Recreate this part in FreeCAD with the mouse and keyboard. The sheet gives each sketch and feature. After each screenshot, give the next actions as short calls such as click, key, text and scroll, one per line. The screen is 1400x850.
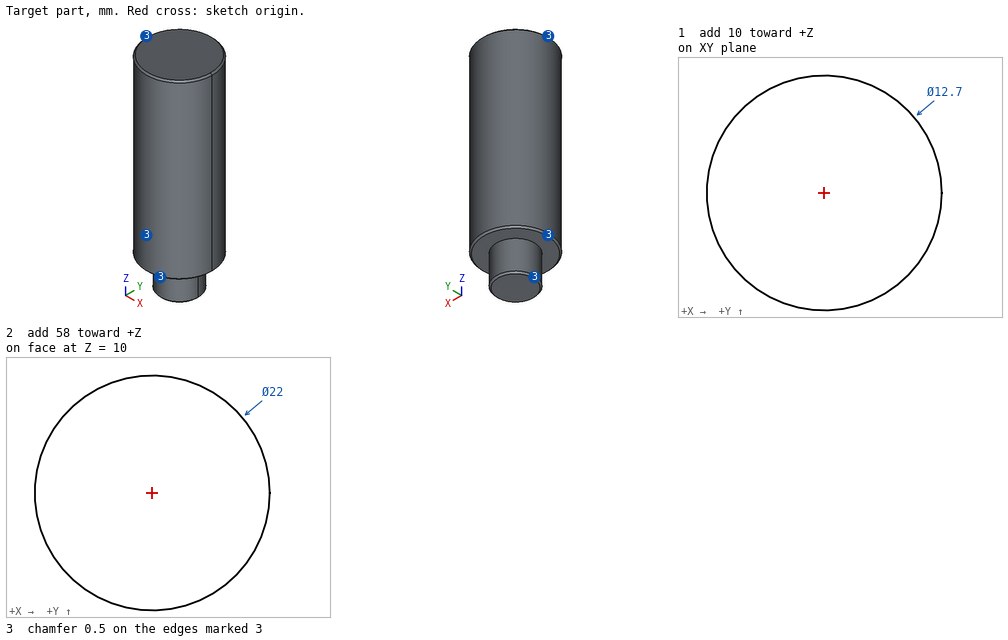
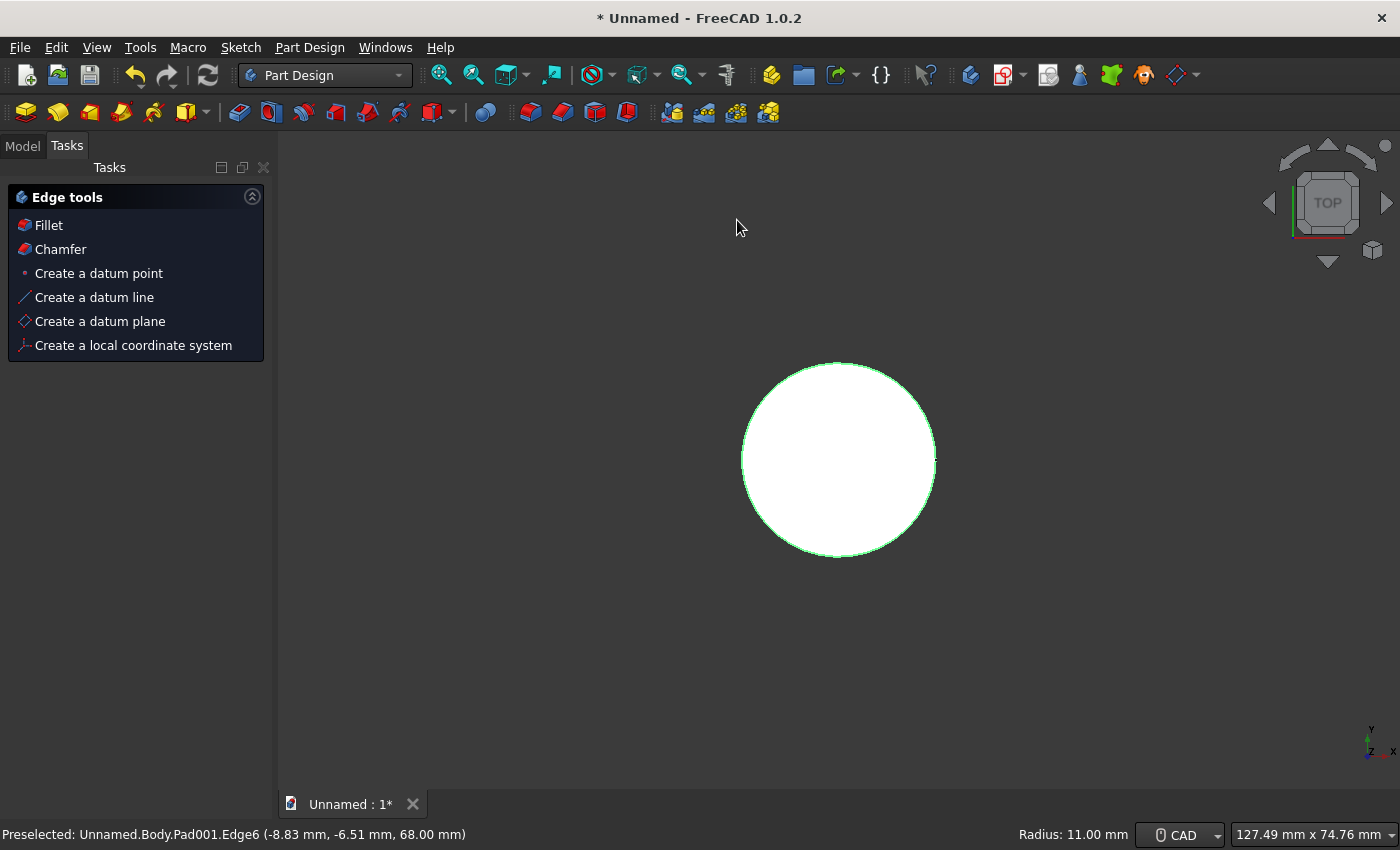
click(442, 76)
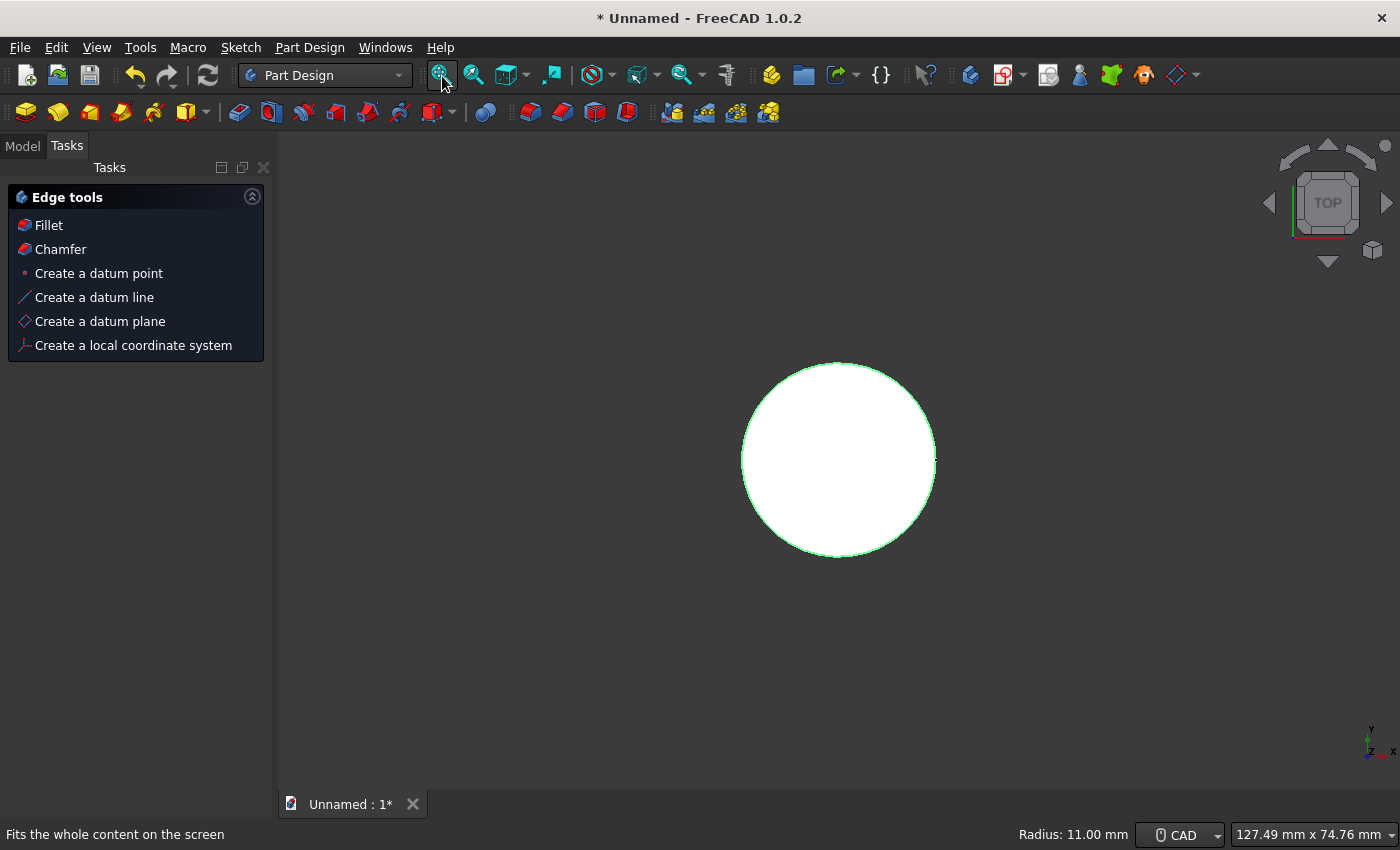
key(1)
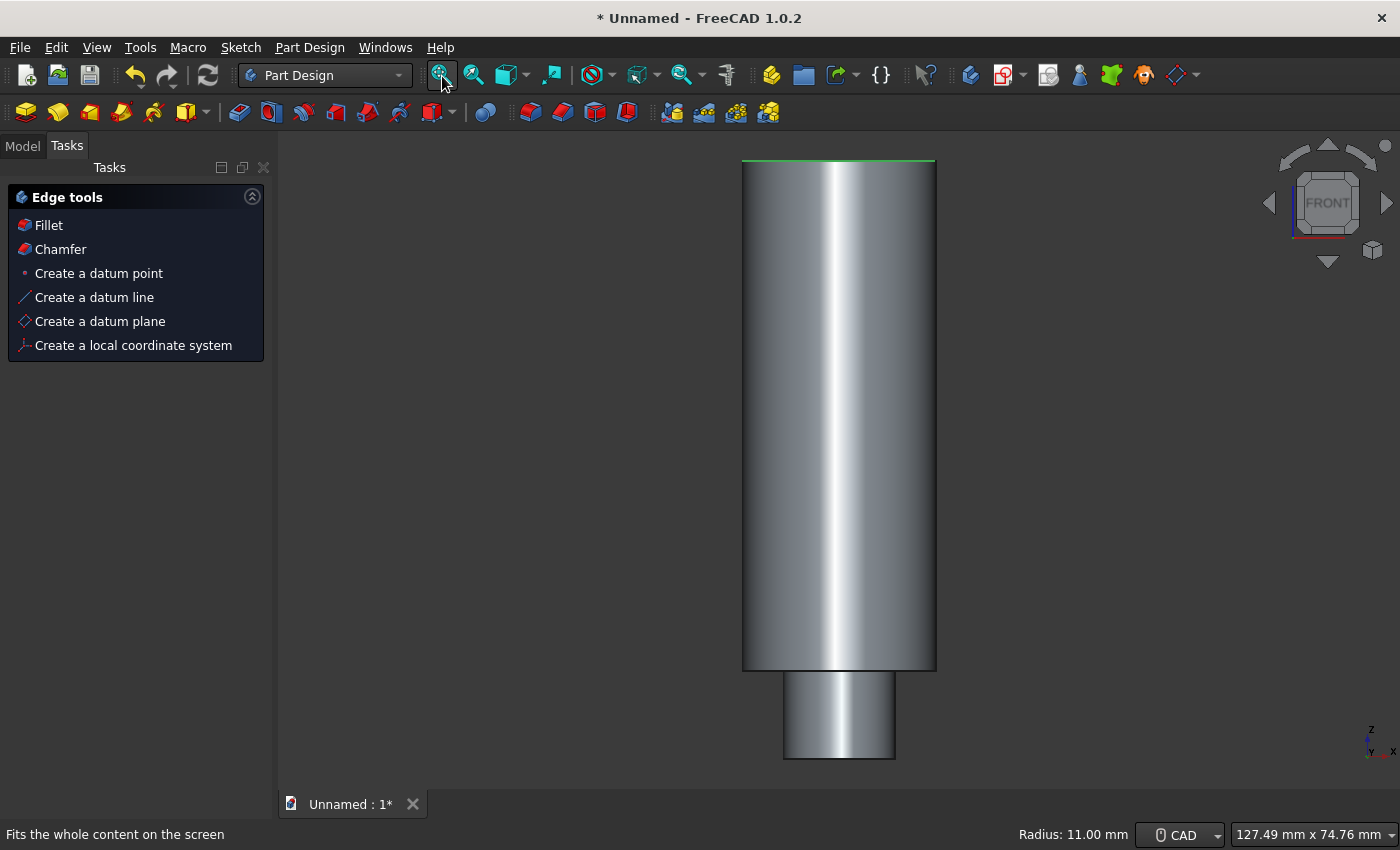
click(794, 758, ctrl)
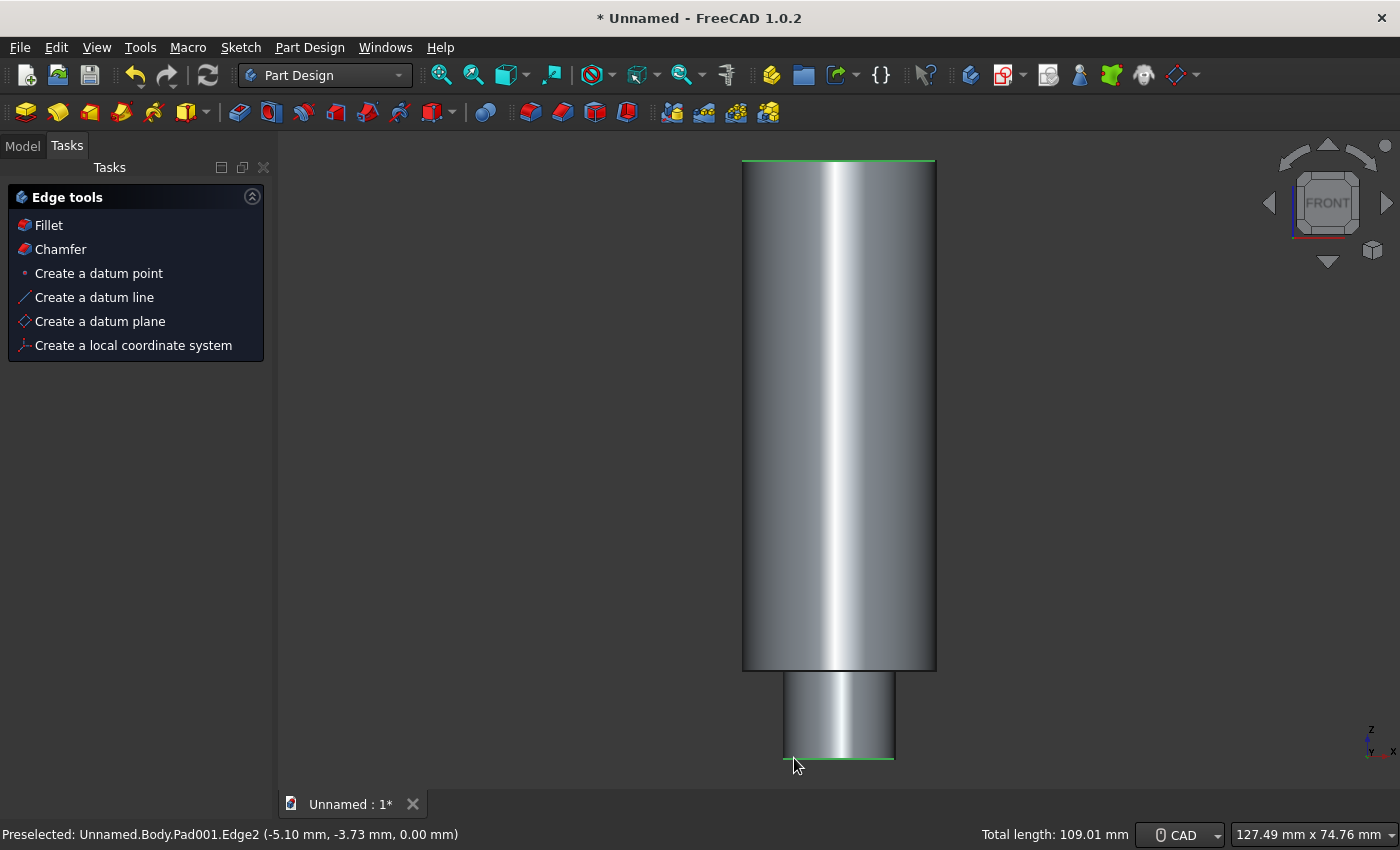
click(761, 670, ctrl)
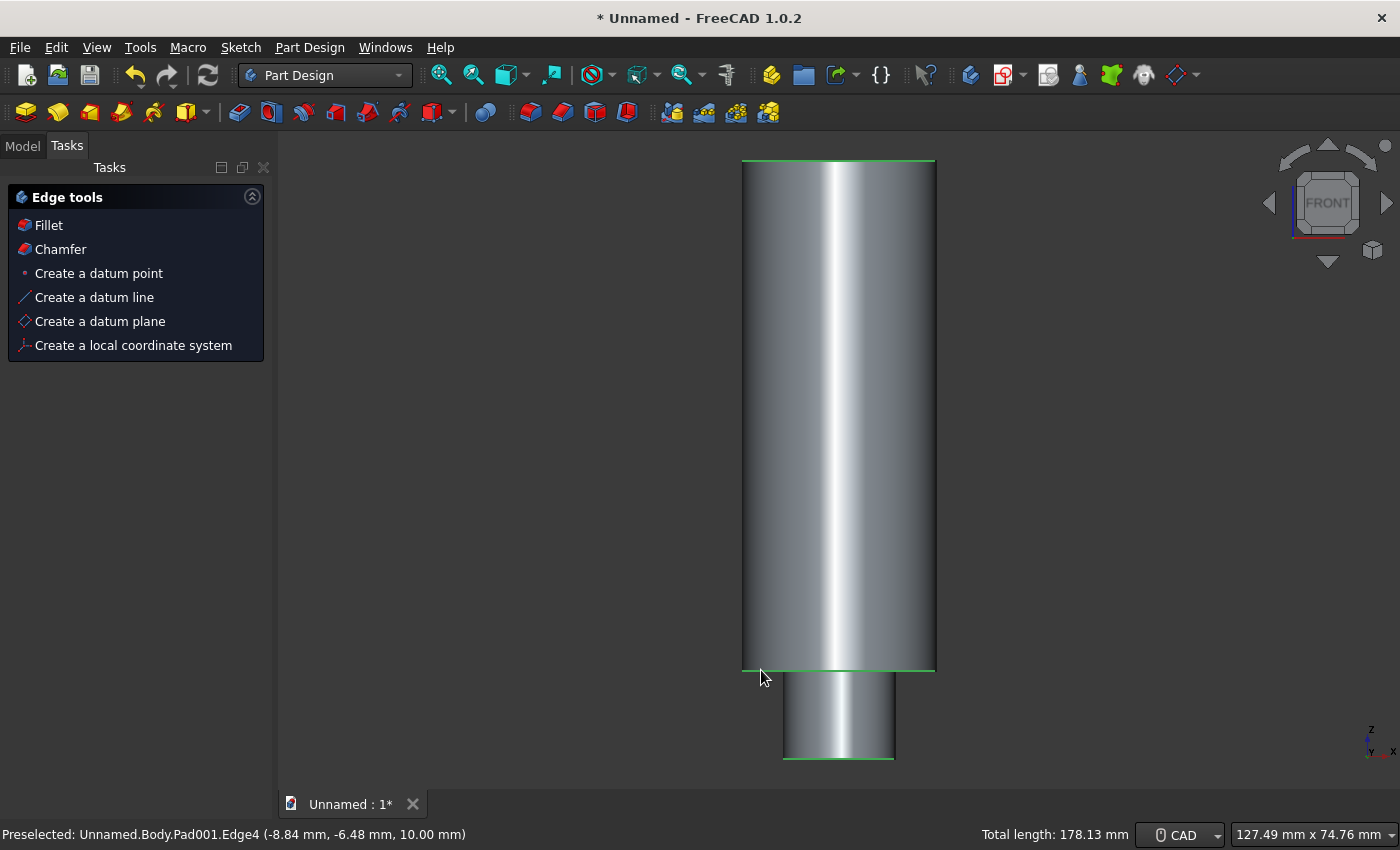
click(564, 112)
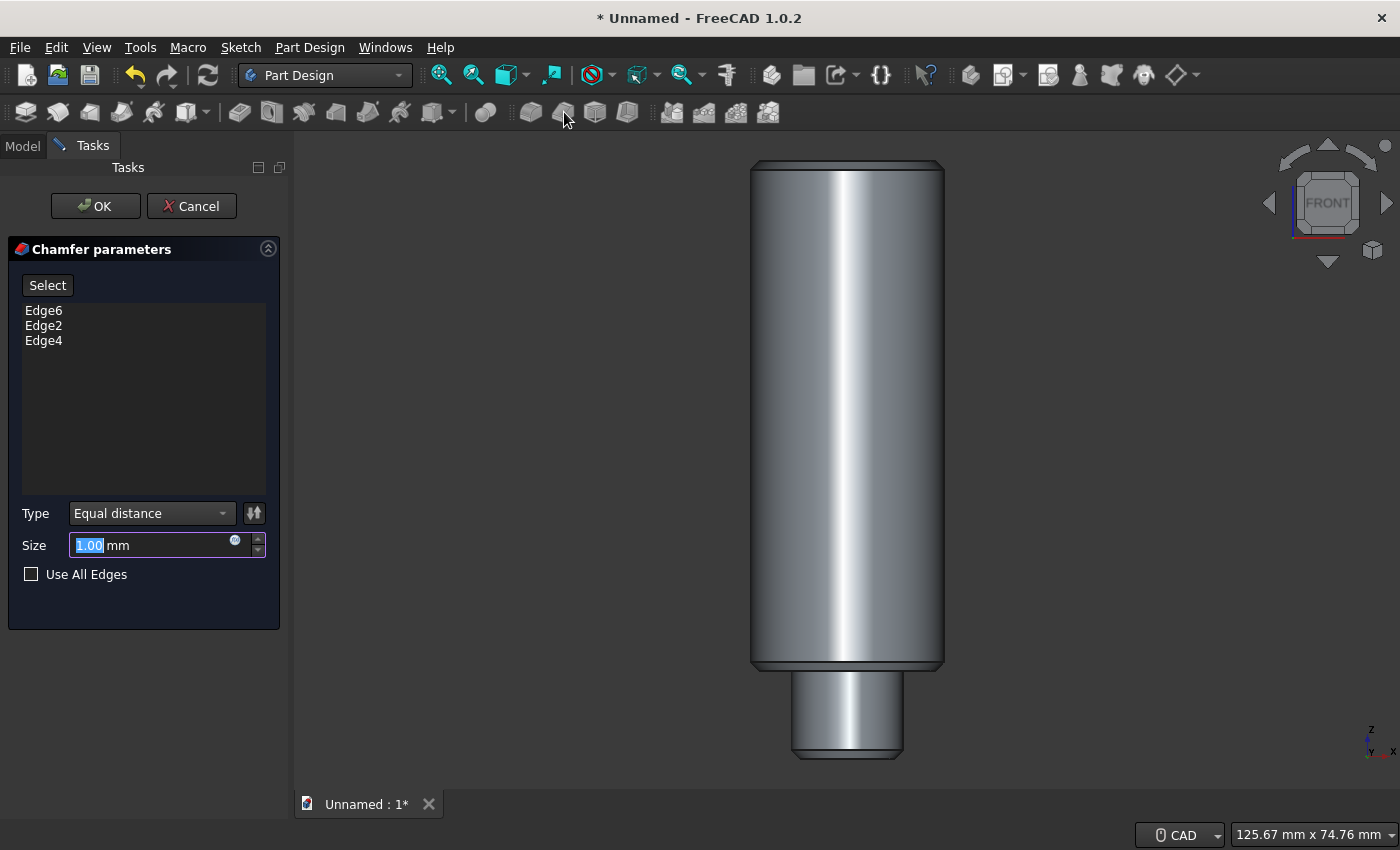
text(0.5)
key(Tab)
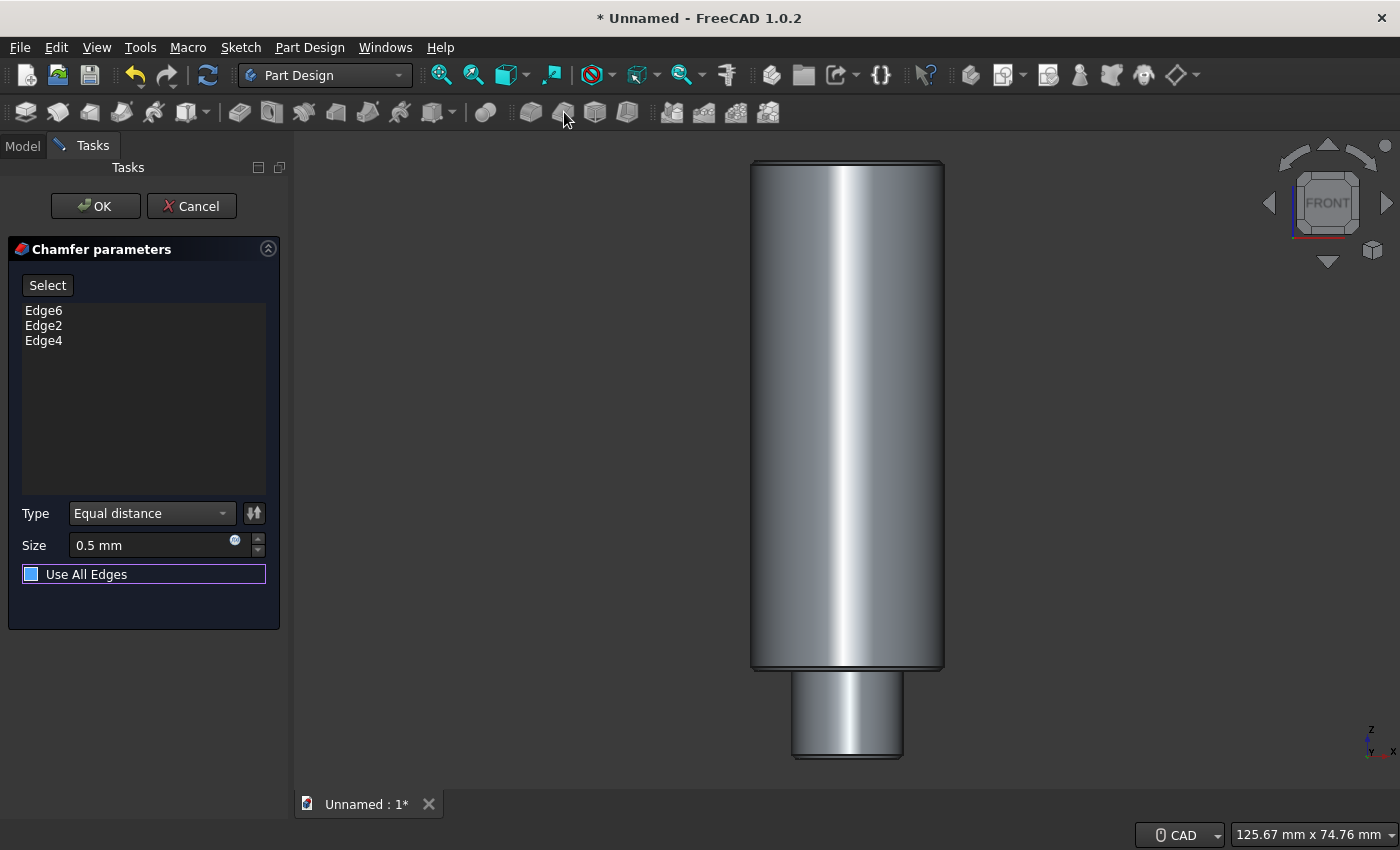
click(96, 206)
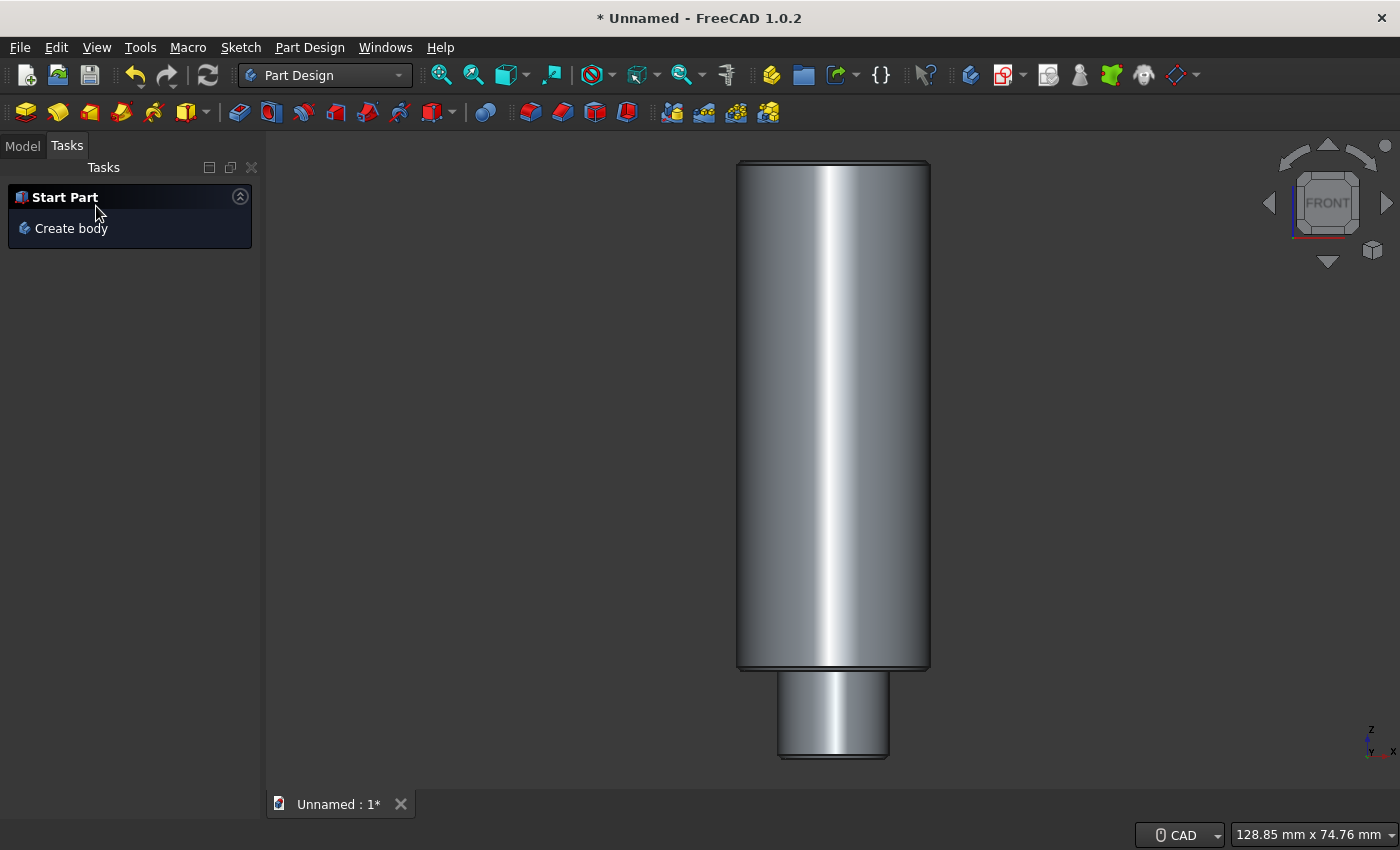
key(0)